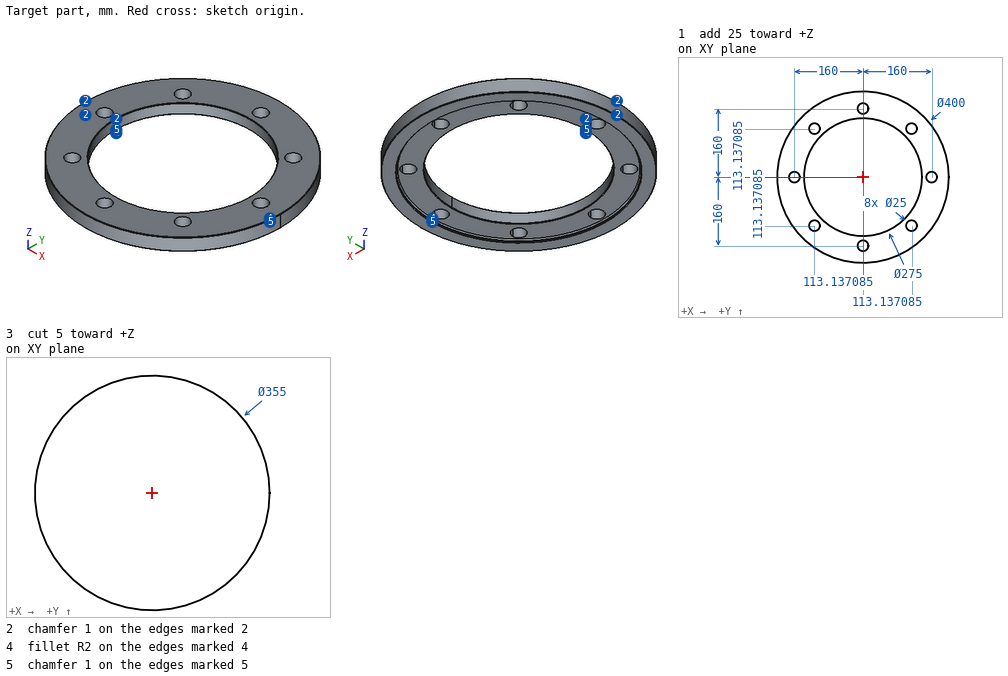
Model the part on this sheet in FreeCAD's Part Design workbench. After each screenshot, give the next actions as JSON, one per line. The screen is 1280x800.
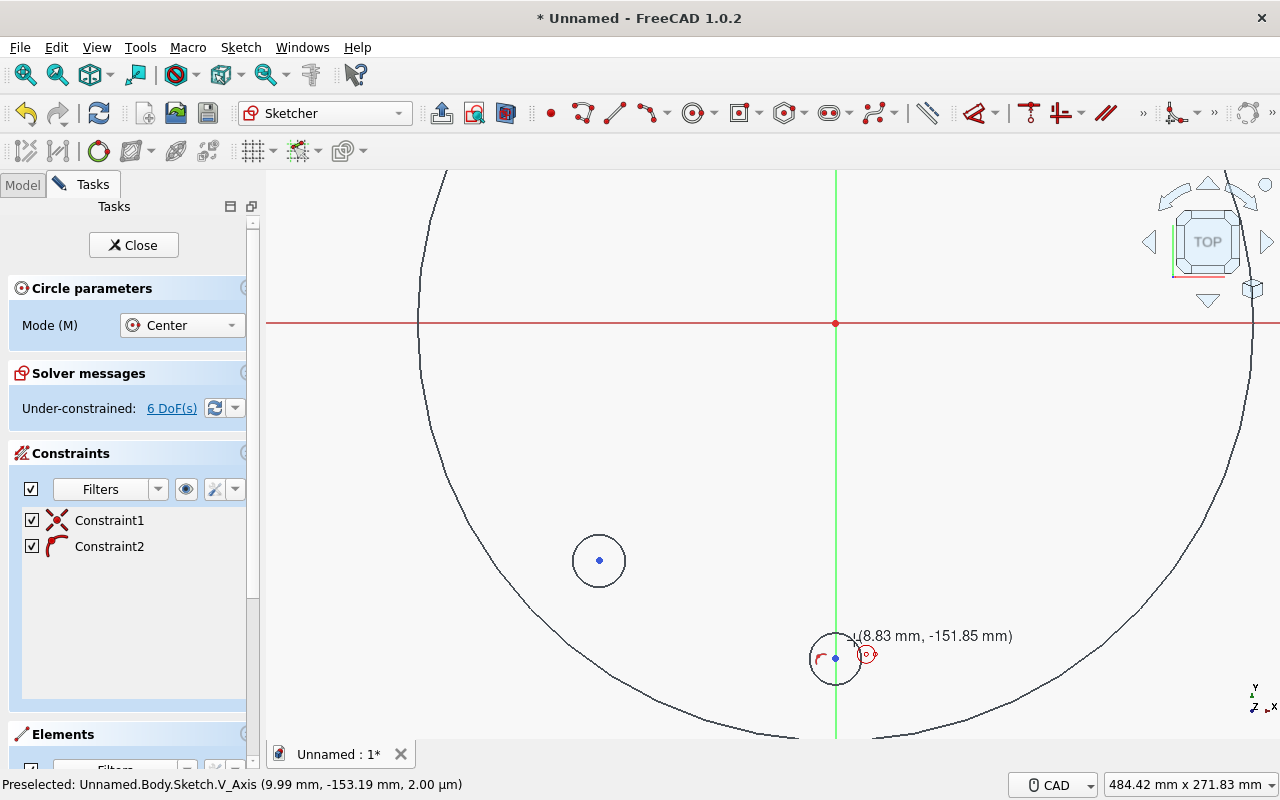
{"action": "left_click", "coordinate": [1072, 560]}
{"action": "left_click", "coordinate": [1091, 541]}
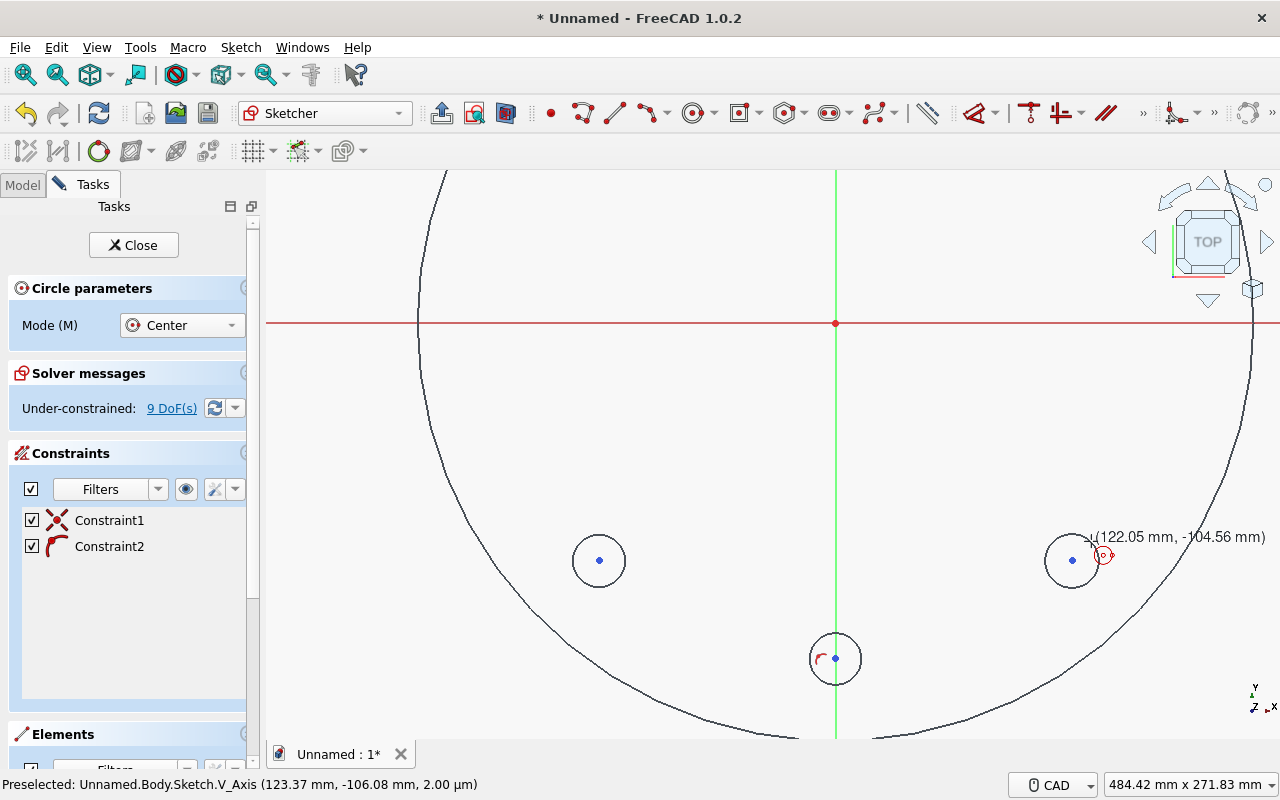
{"action": "left_click", "coordinate": [501, 323]}
{"action": "left_click", "coordinate": [519, 305]}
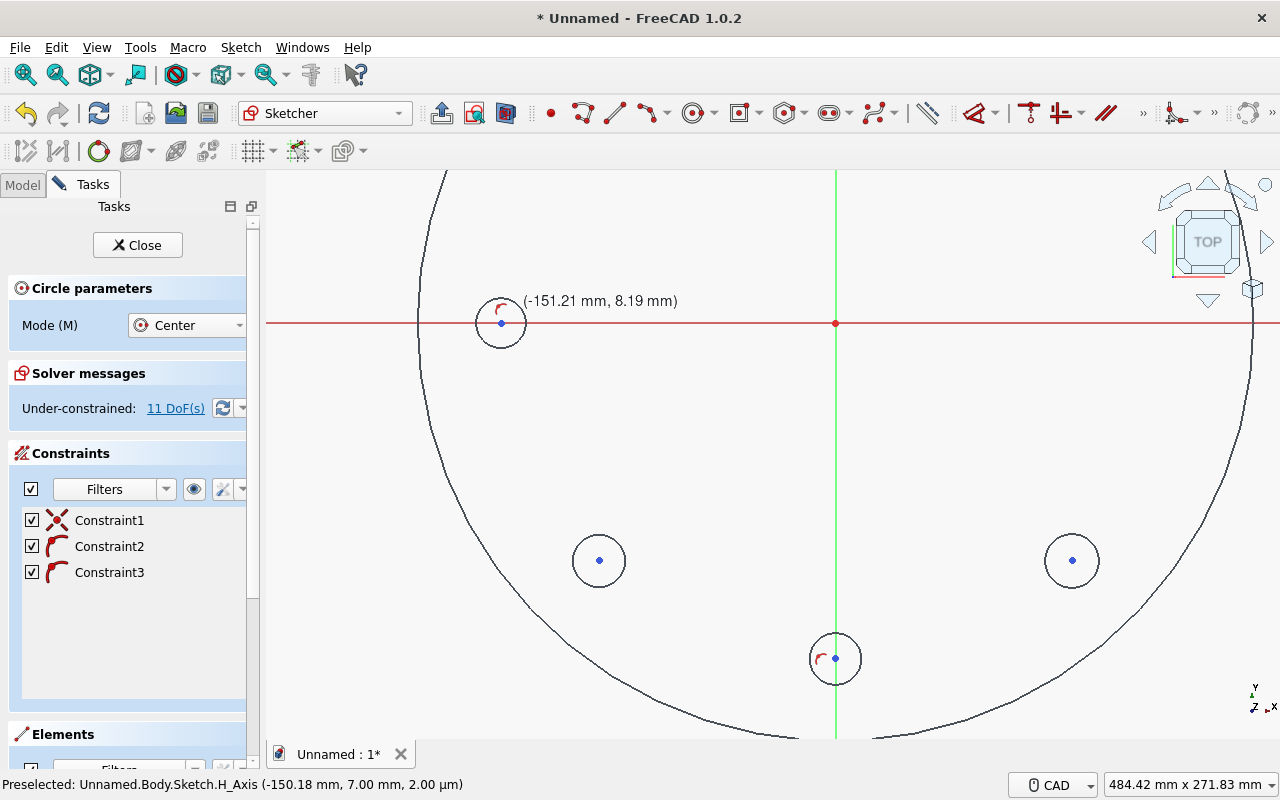
{"action": "scroll", "coordinate": [598, 562], "scroll_direction": "down", "scroll_amount": 4}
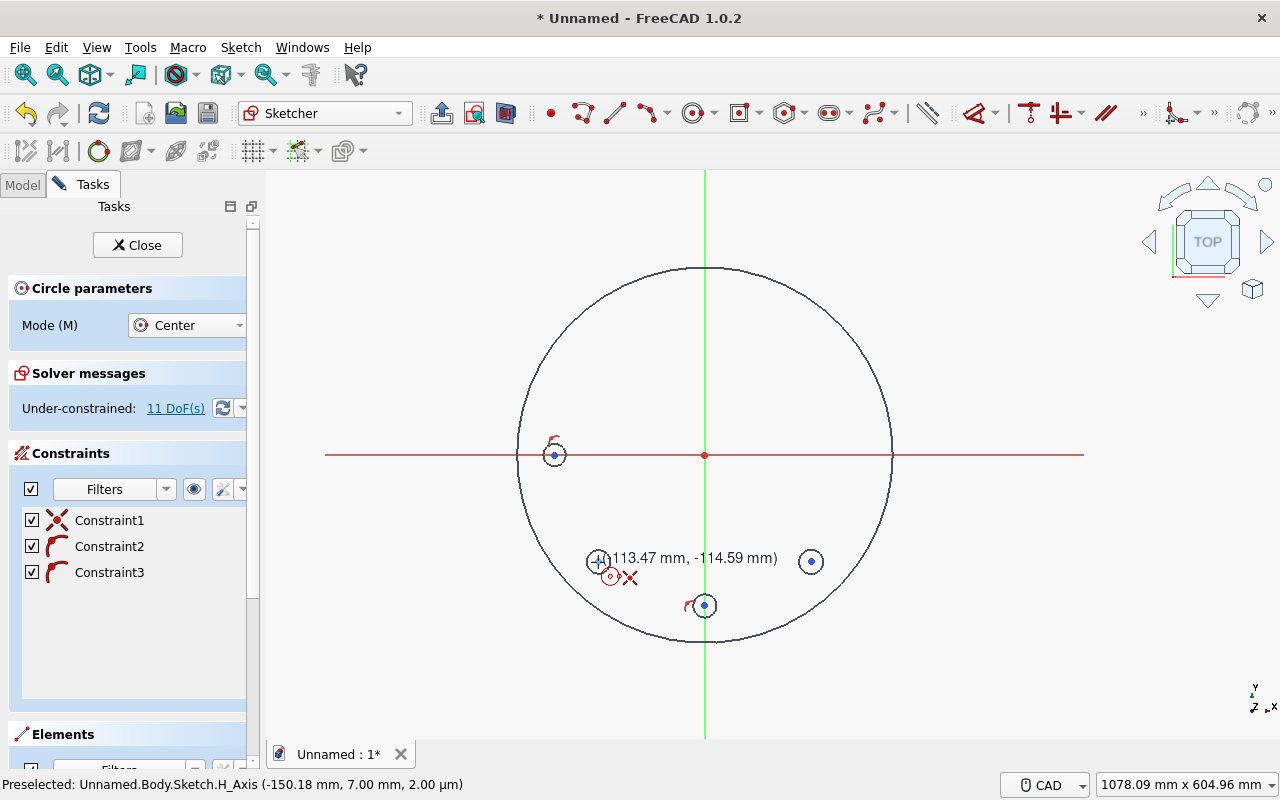
{"action": "scroll", "coordinate": [598, 349], "scroll_direction": "up", "scroll_amount": 4}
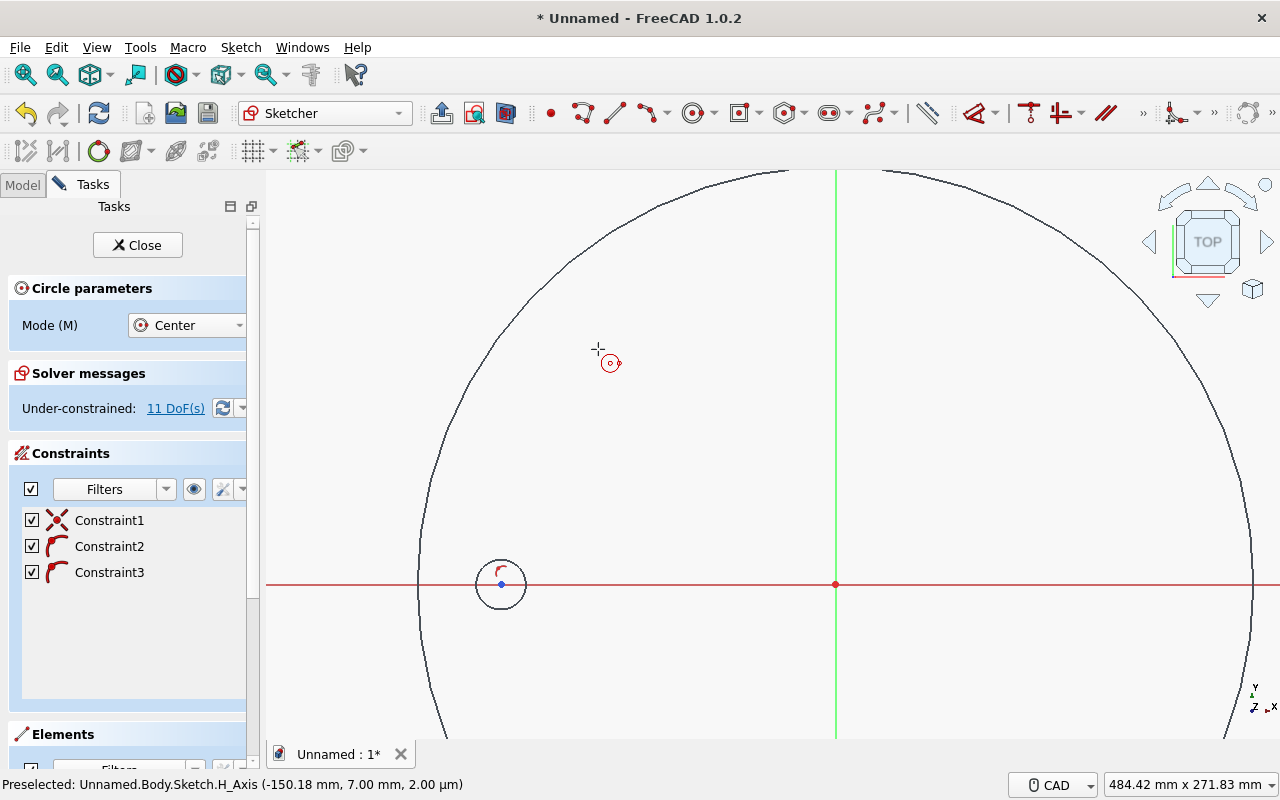
{"action": "left_click", "coordinate": [599, 348]}
{"action": "left_click", "coordinate": [617, 329]}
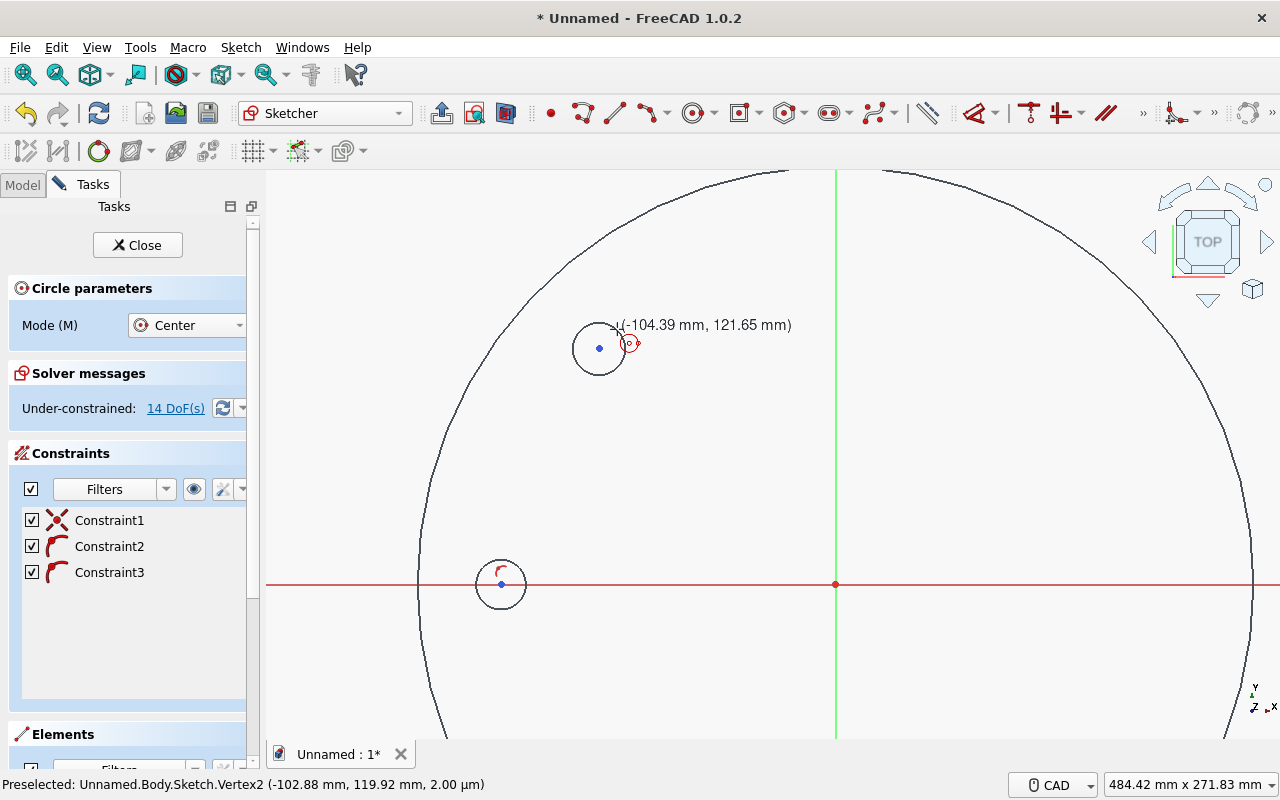
{"action": "left_click", "coordinate": [836, 585]}
{"action": "left_click", "coordinate": [1039, 381]}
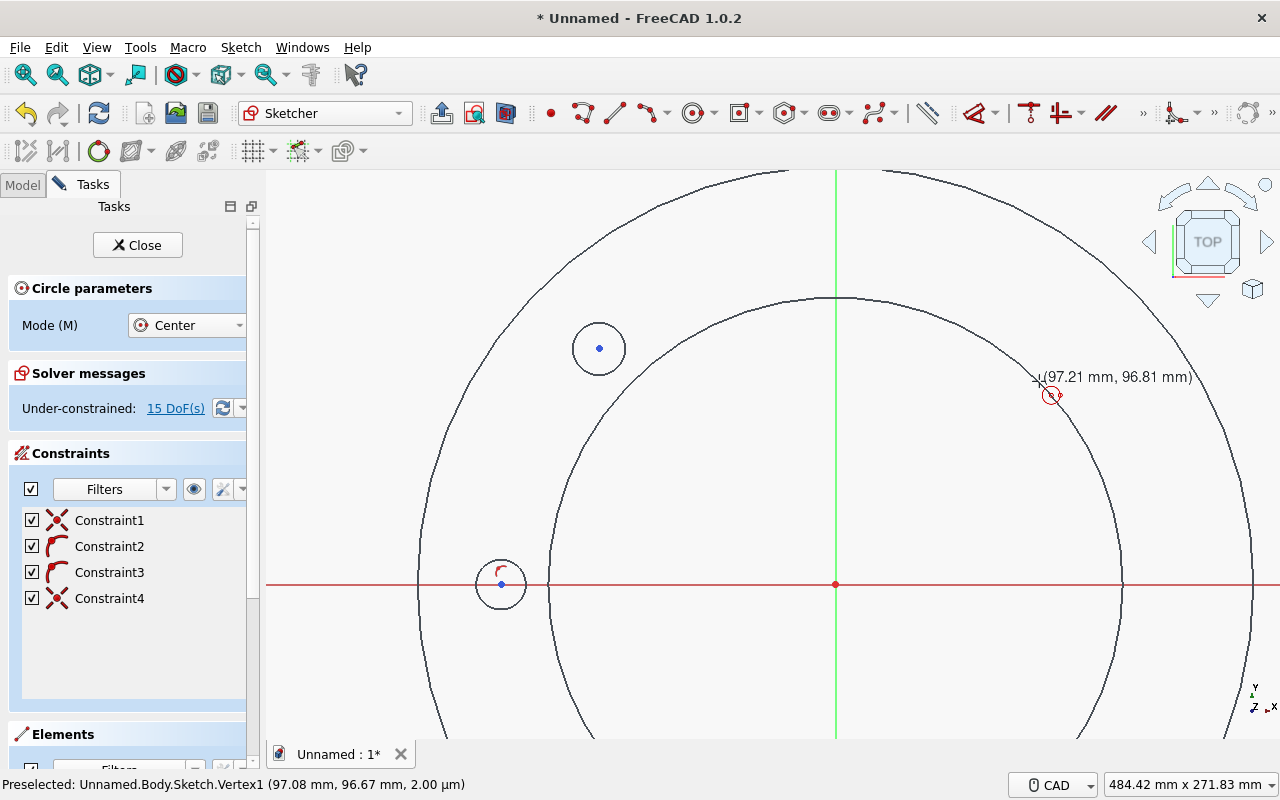
{"action": "scroll", "coordinate": [598, 348], "scroll_direction": "down", "scroll_amount": 4}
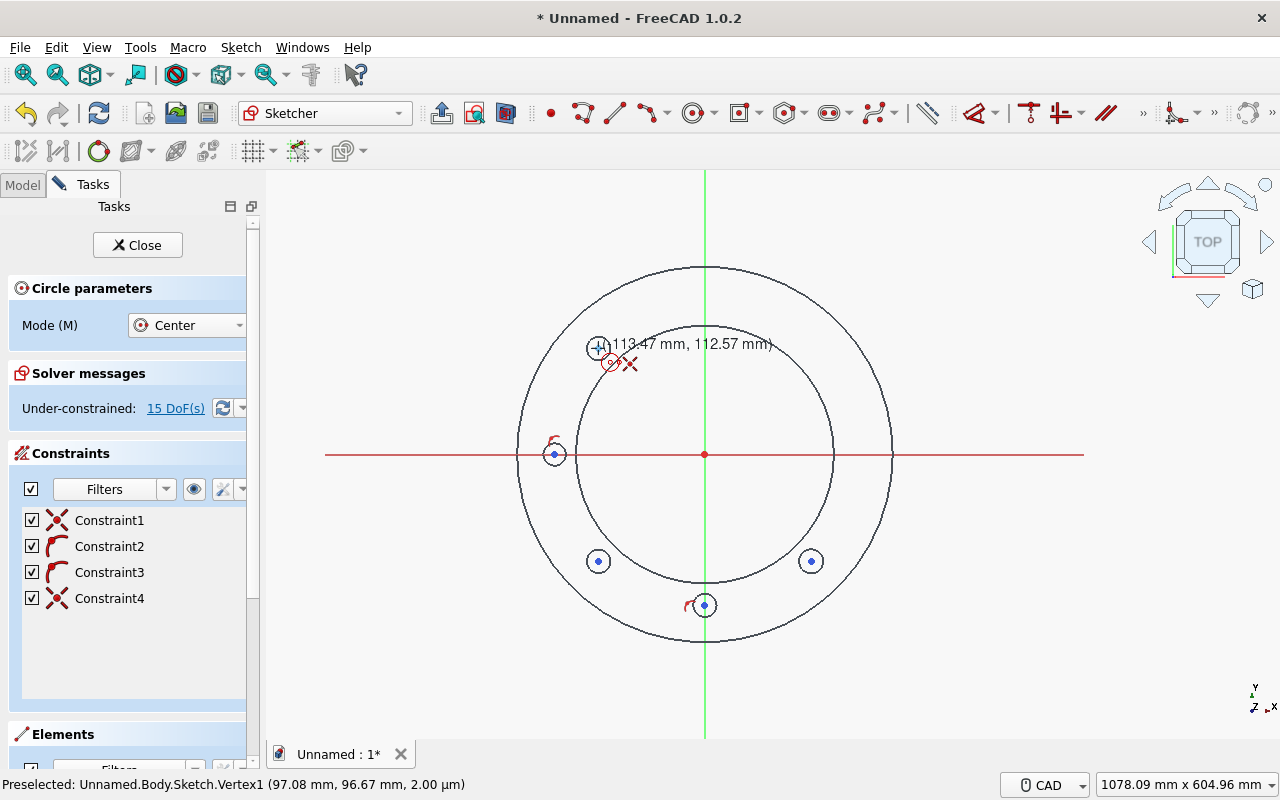
{"action": "scroll", "coordinate": [855, 454], "scroll_direction": "up", "scroll_amount": 4}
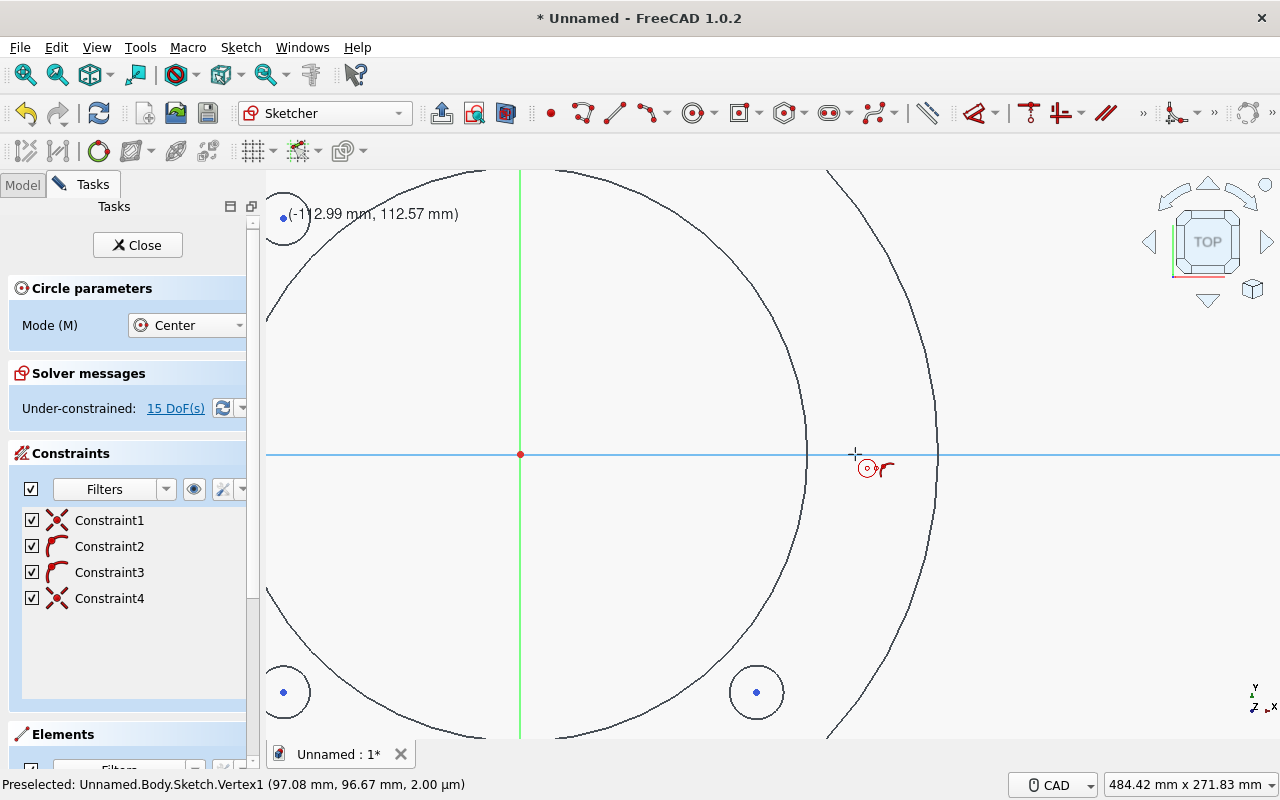
{"action": "left_click", "coordinate": [855, 454]}
{"action": "left_click", "coordinate": [874, 436]}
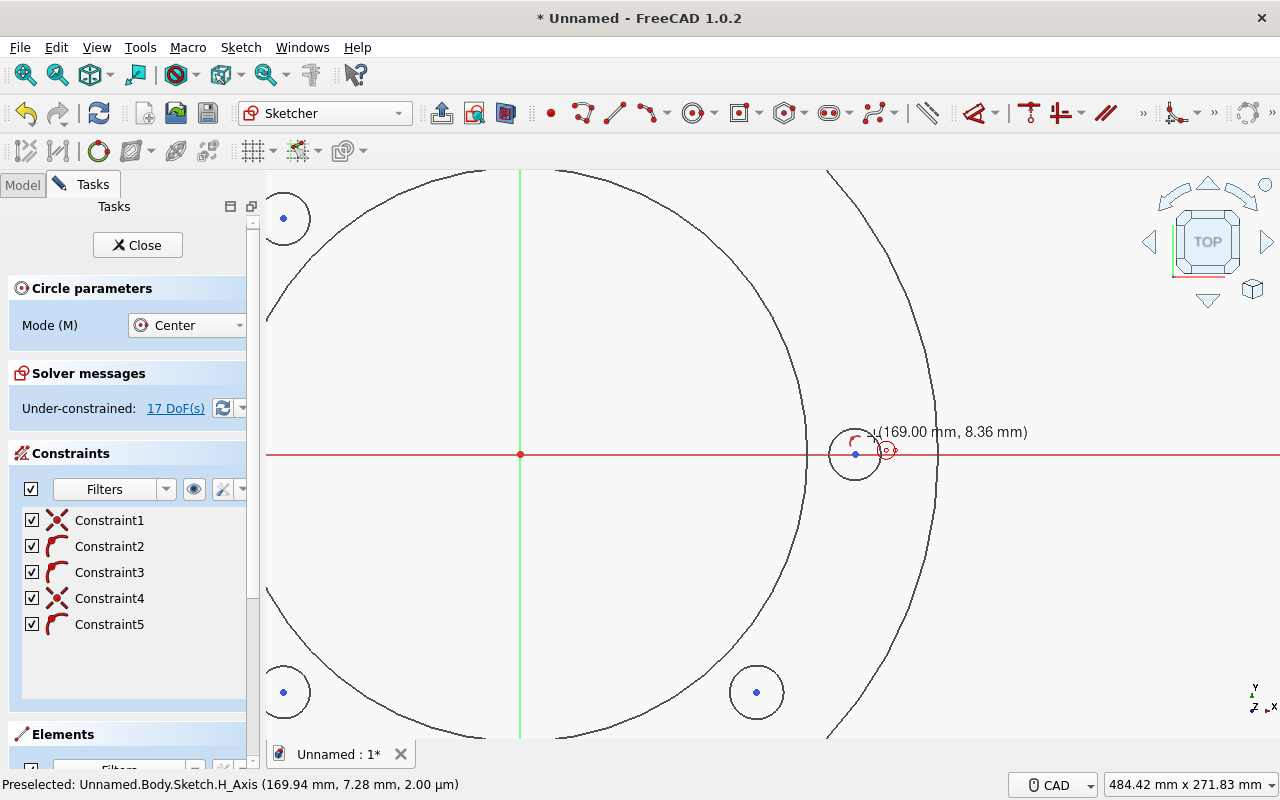
{"action": "scroll", "coordinate": [855, 454], "scroll_direction": "down", "scroll_amount": 4}